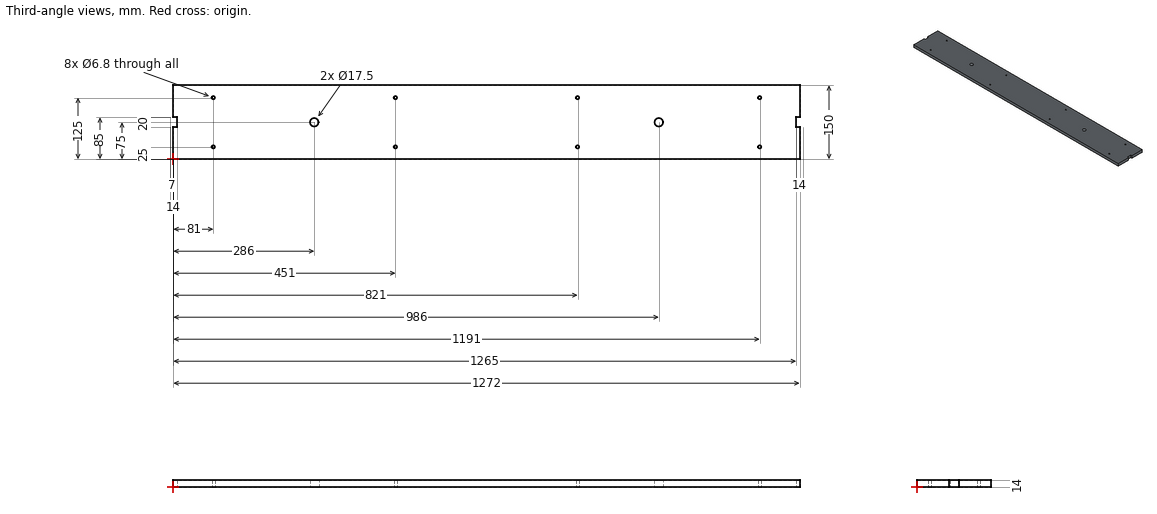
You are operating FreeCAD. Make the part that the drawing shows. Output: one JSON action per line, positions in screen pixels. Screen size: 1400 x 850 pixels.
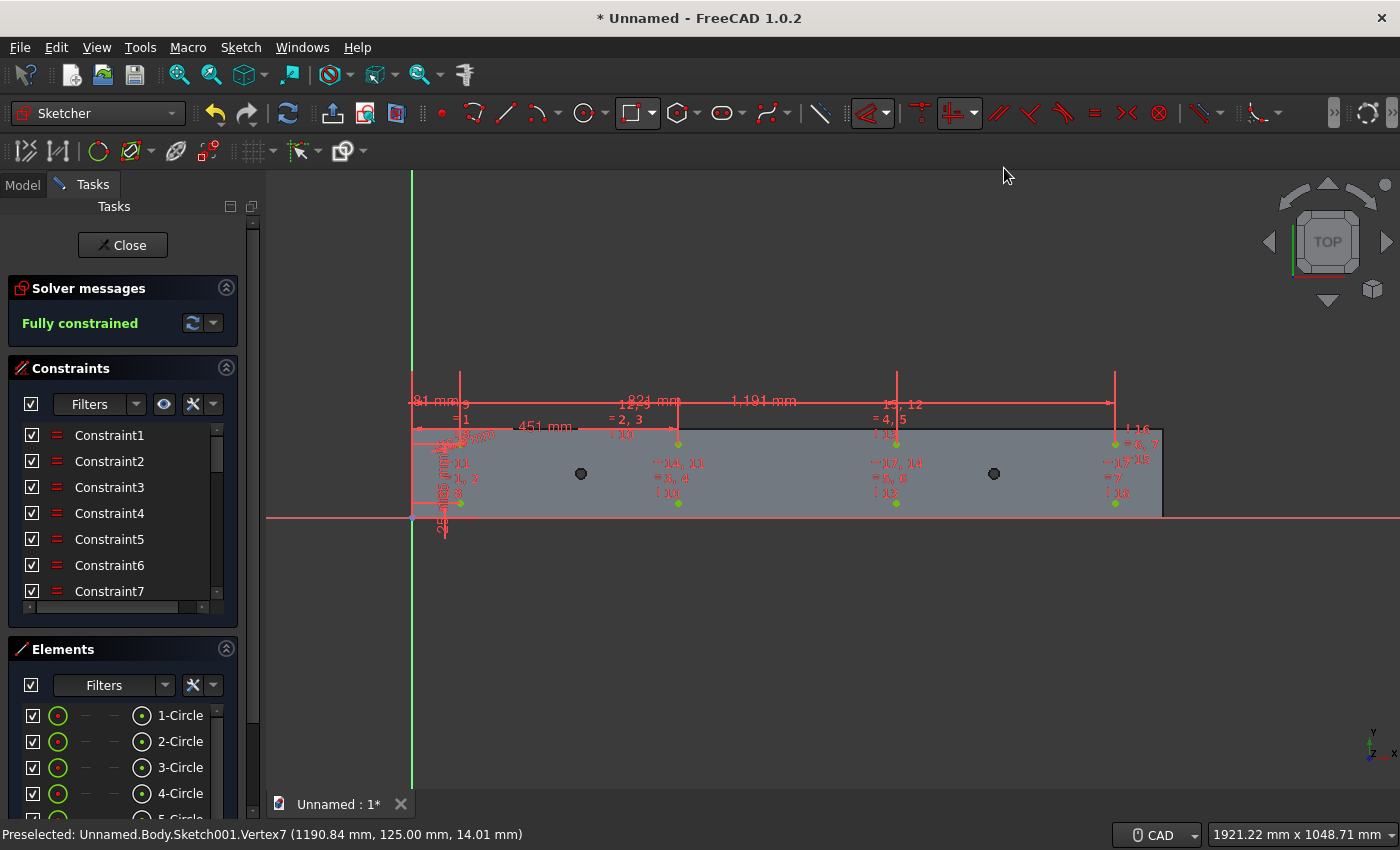
{"action": "left_click", "coordinate": [123, 245]}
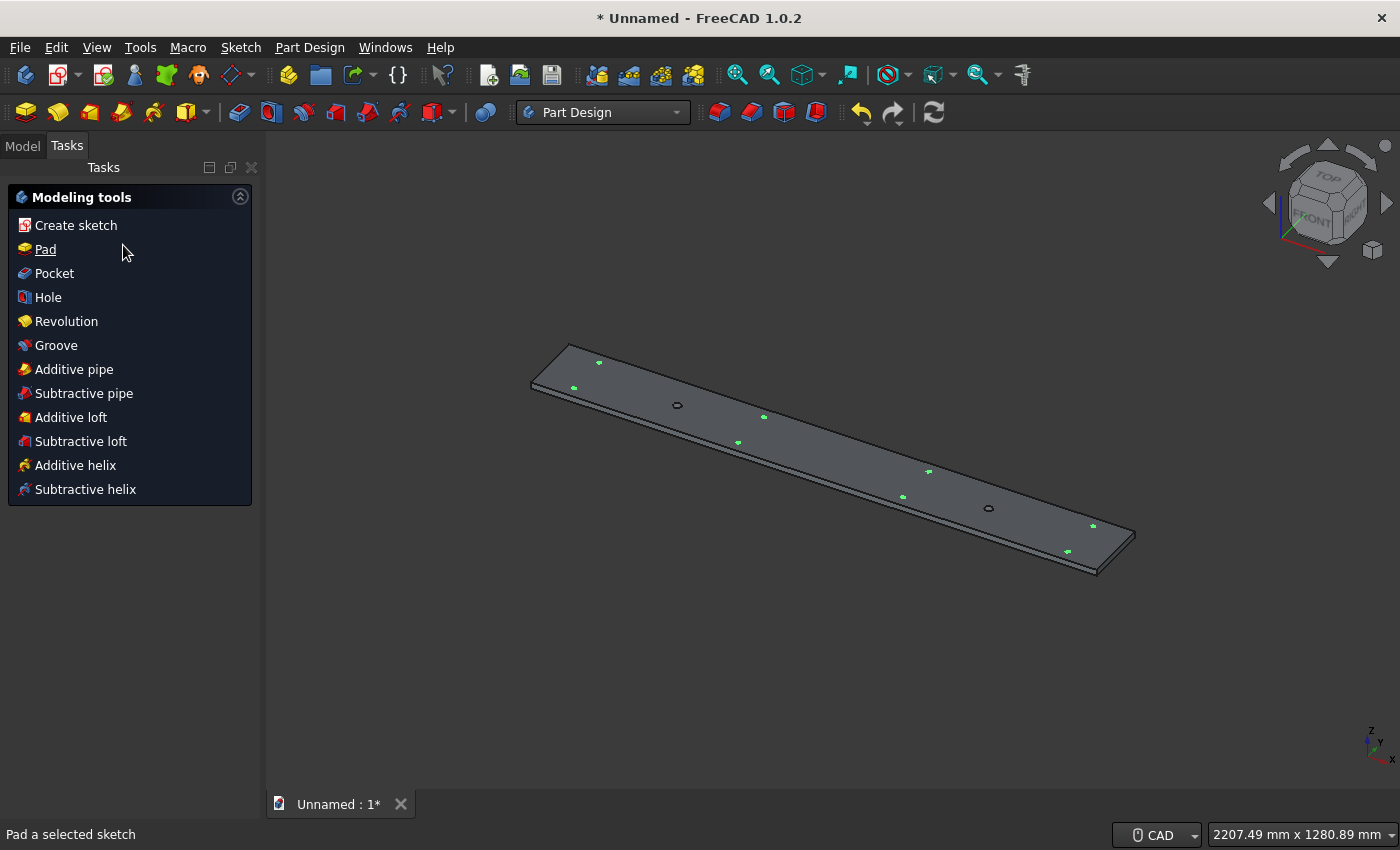
{"action": "left_click", "coordinate": [272, 112]}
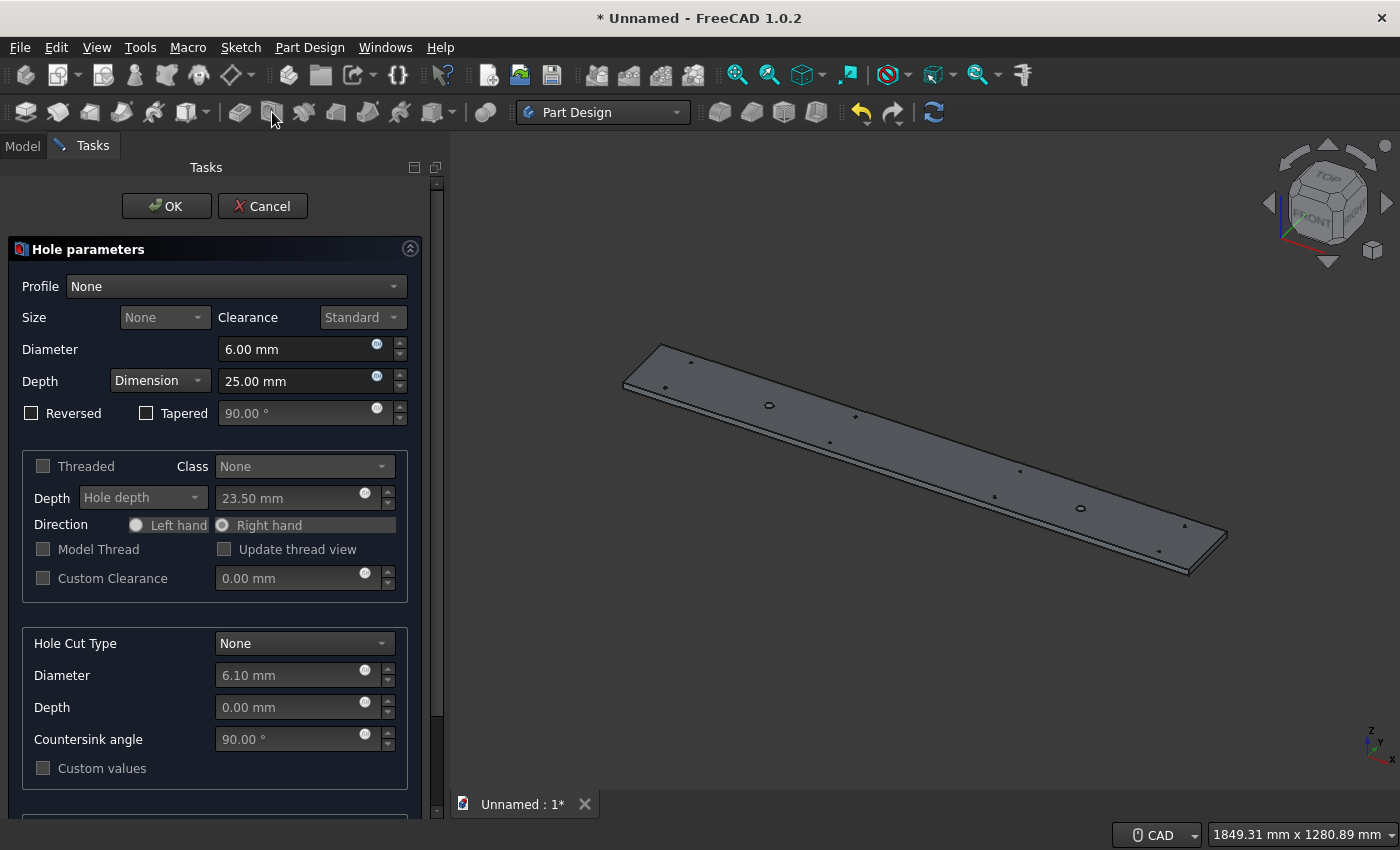
{"action": "triple_click", "coordinate": [305, 349]}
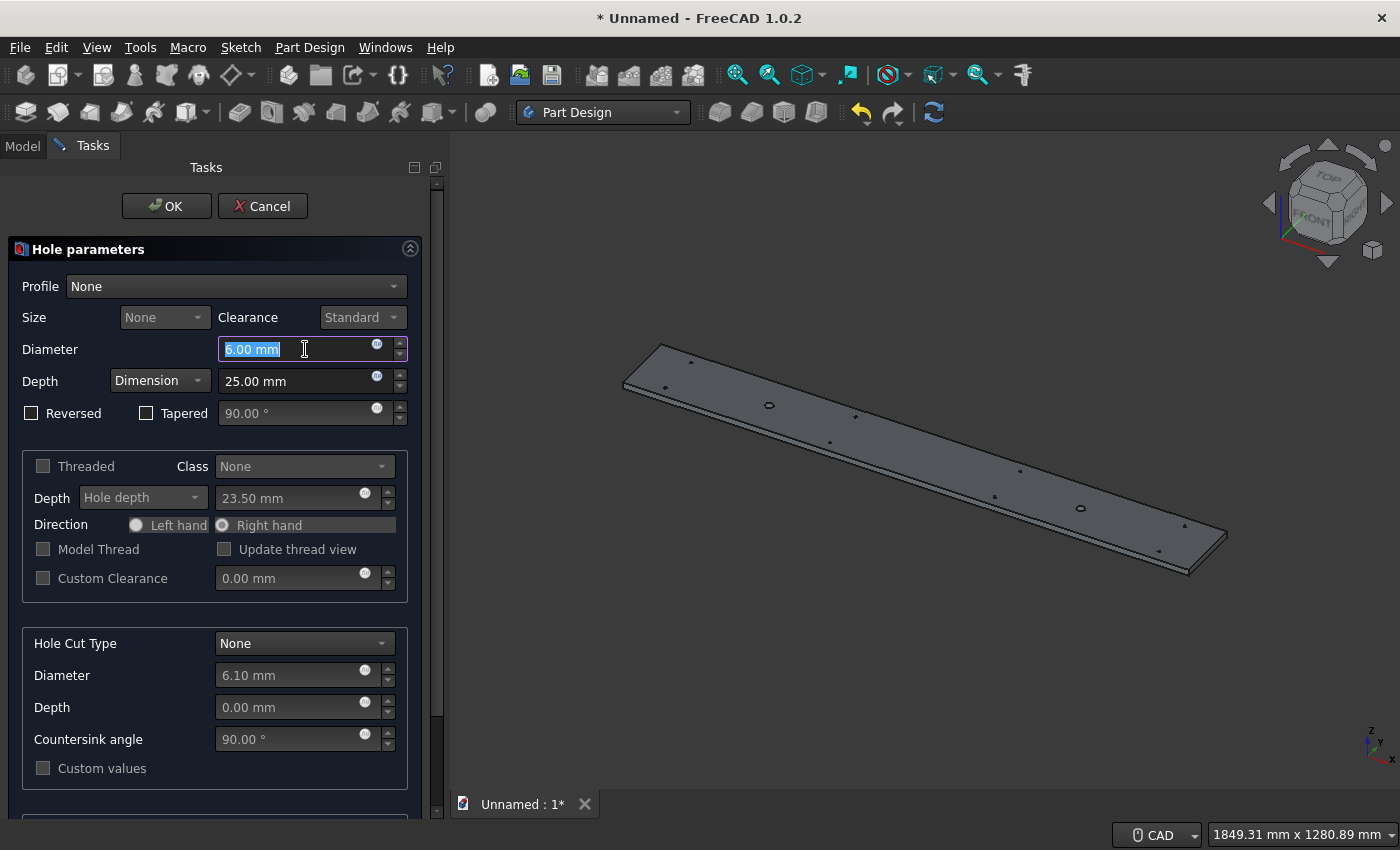
{"action": "type", "text": "6.8"}
{"action": "key", "text": "Tab"}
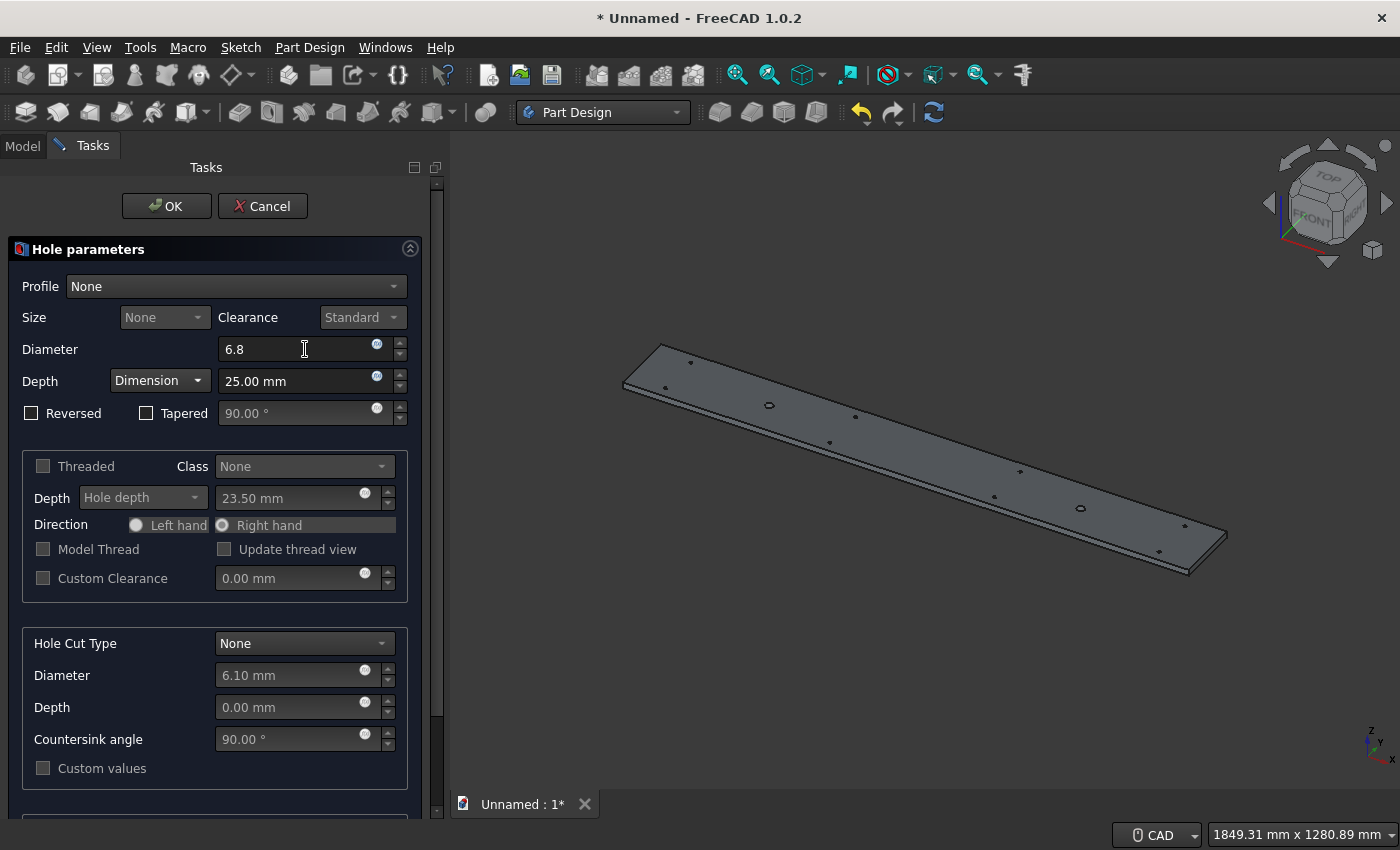
{"action": "left_click", "coordinate": [161, 380]}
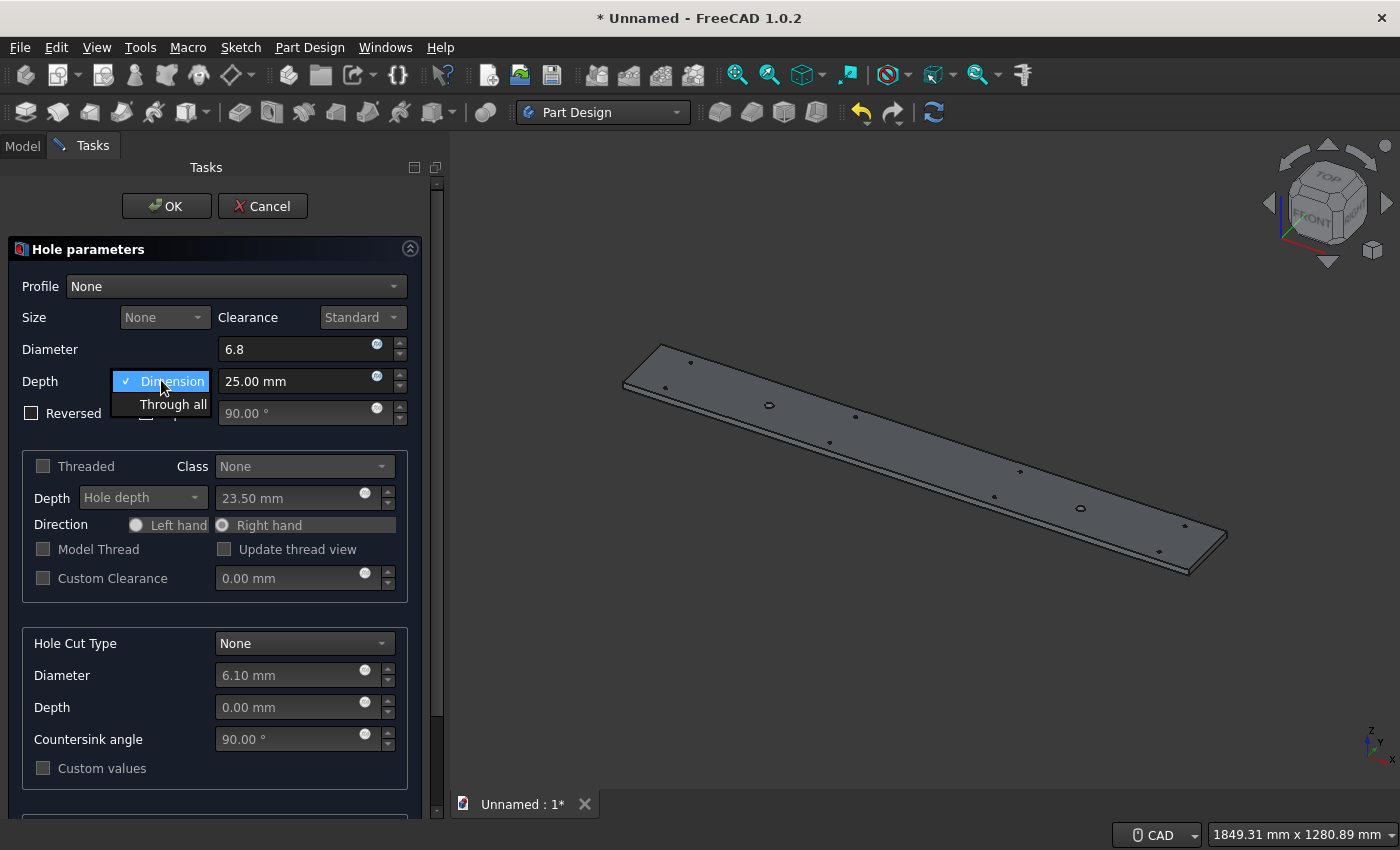
{"action": "left_click", "coordinate": [160, 404]}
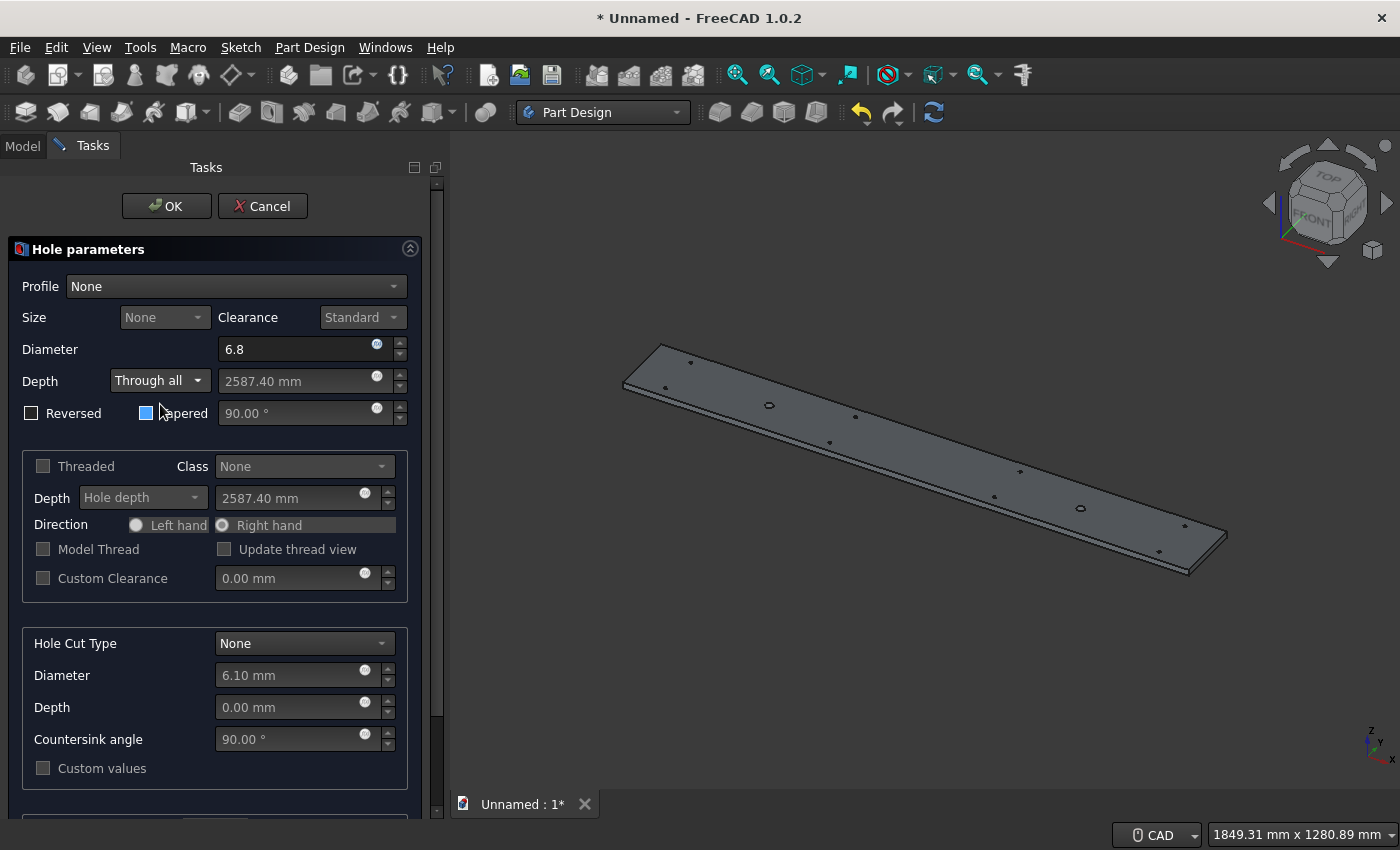
{"action": "left_click", "coordinate": [167, 206]}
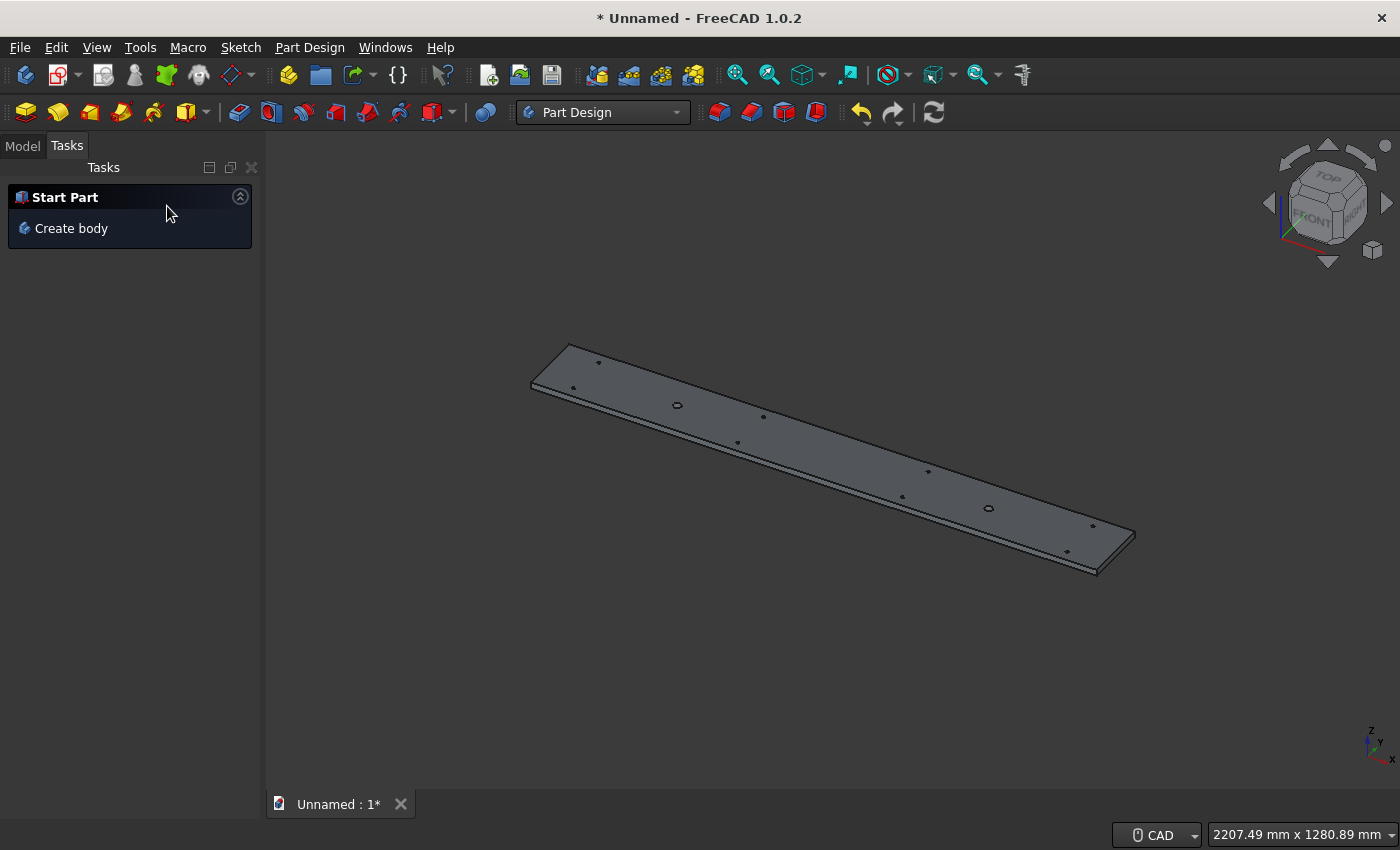
{"action": "left_click", "coordinate": [833, 456]}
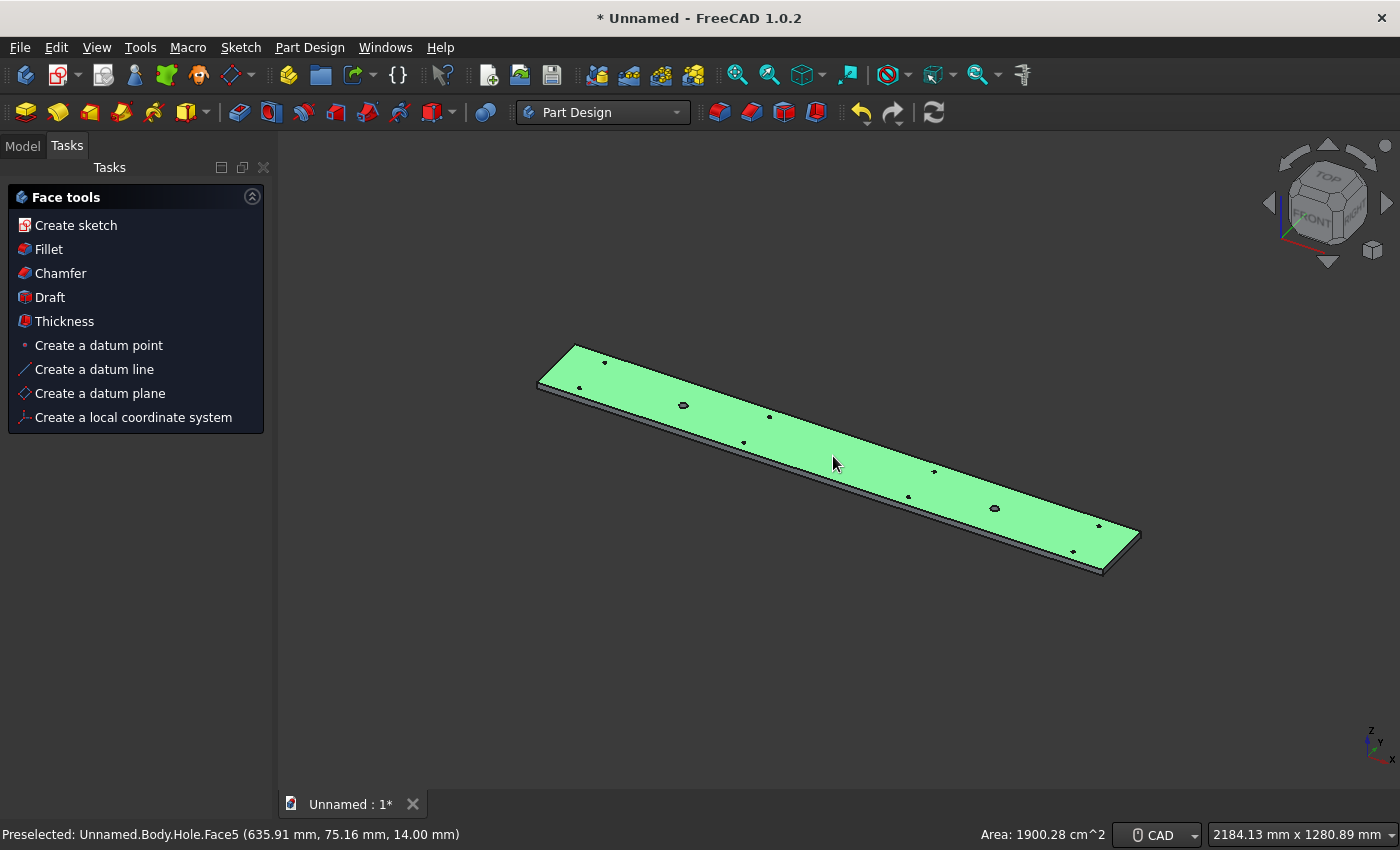
{"action": "left_click", "coordinate": [58, 76]}